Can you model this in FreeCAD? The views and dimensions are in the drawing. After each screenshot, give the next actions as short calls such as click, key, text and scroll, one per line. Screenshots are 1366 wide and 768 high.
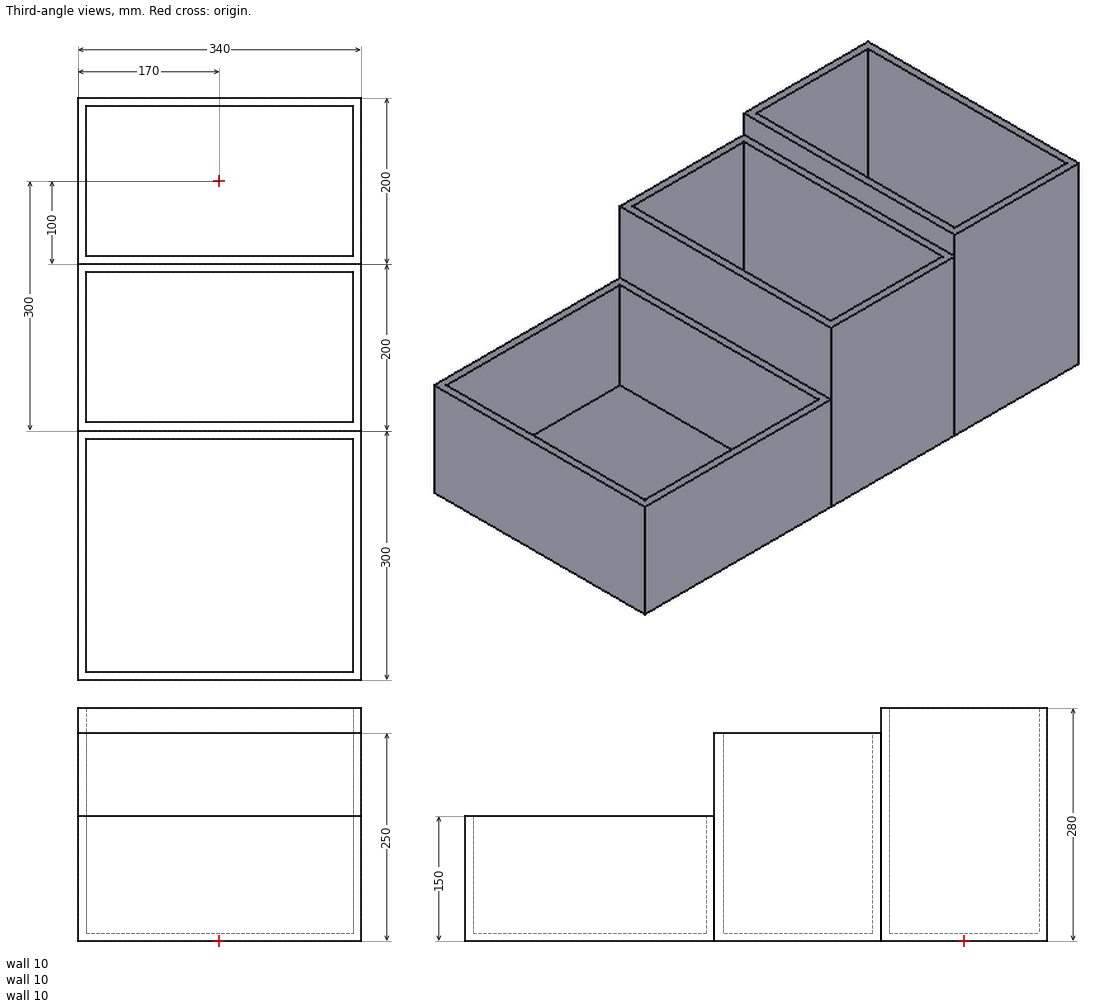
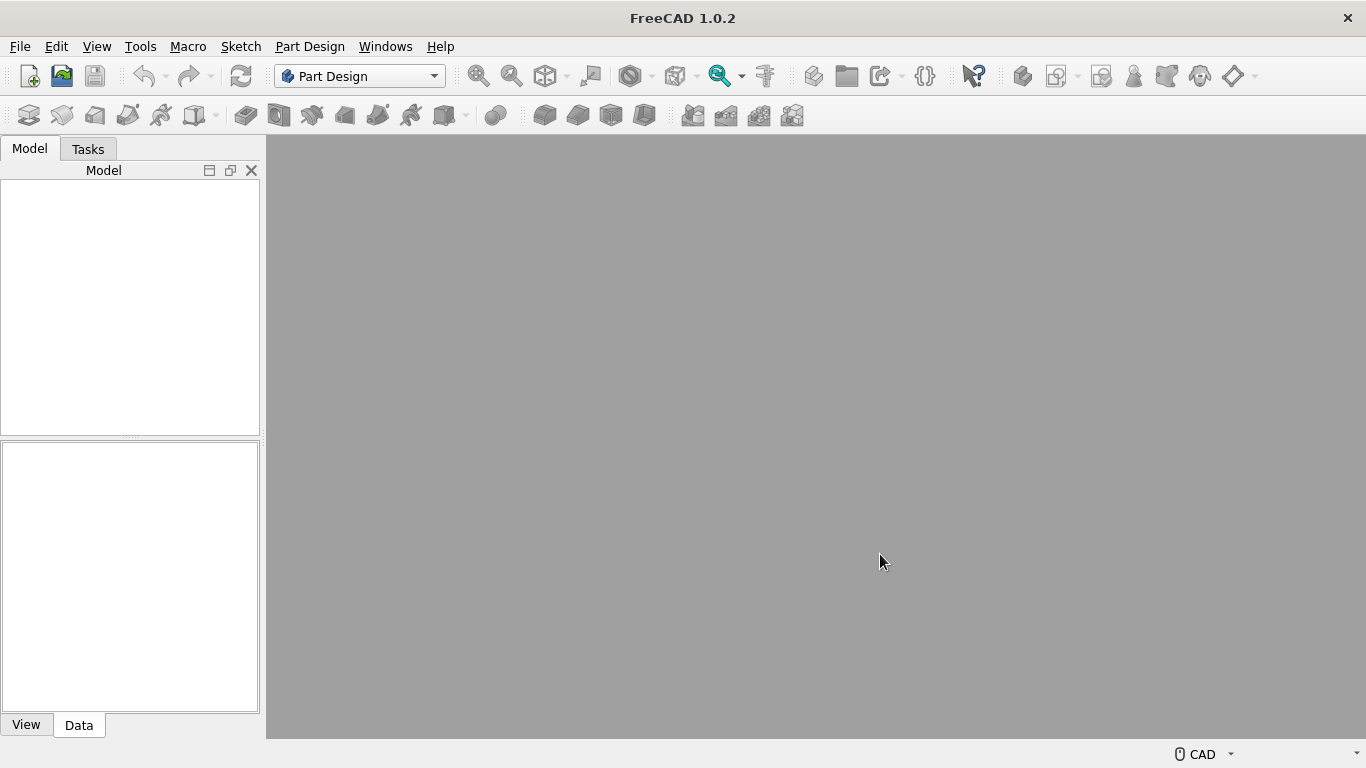
key(ctrl+n)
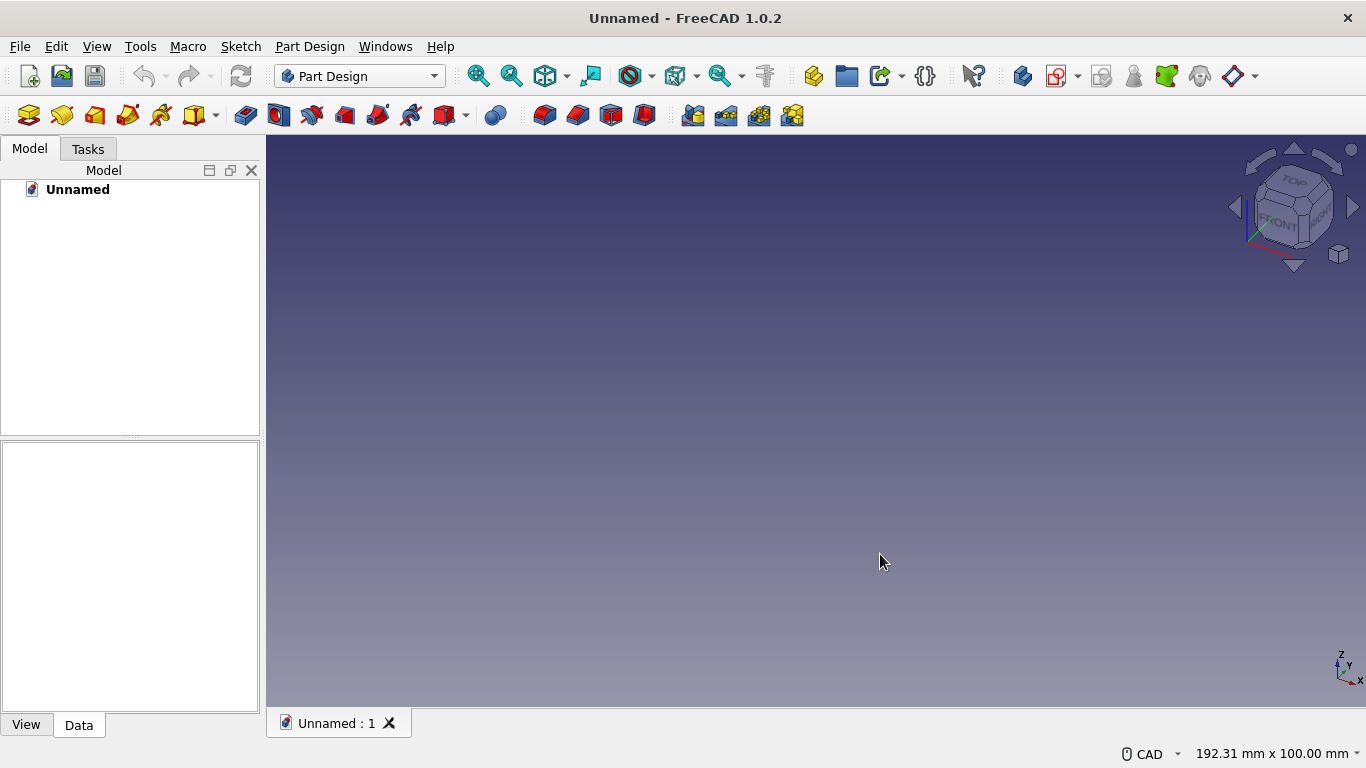
click(1056, 76)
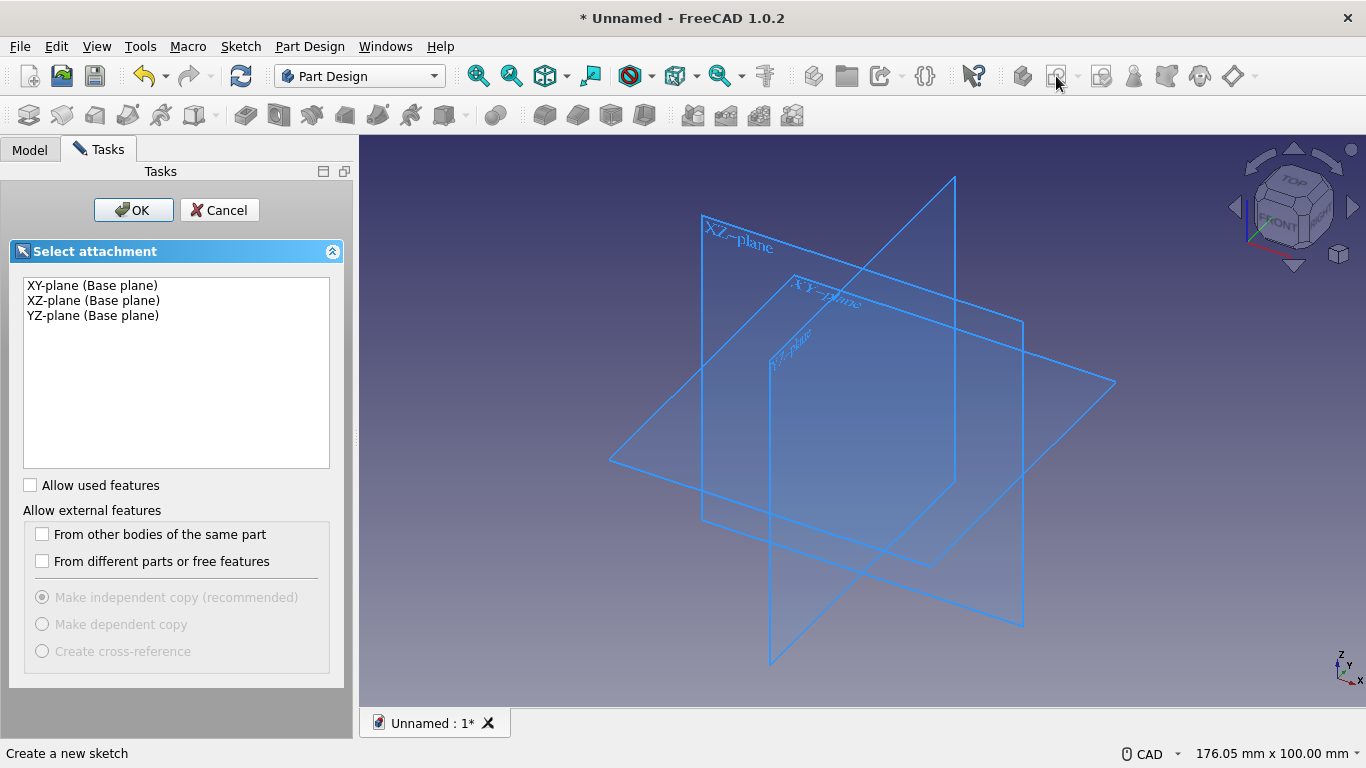
click(84, 286)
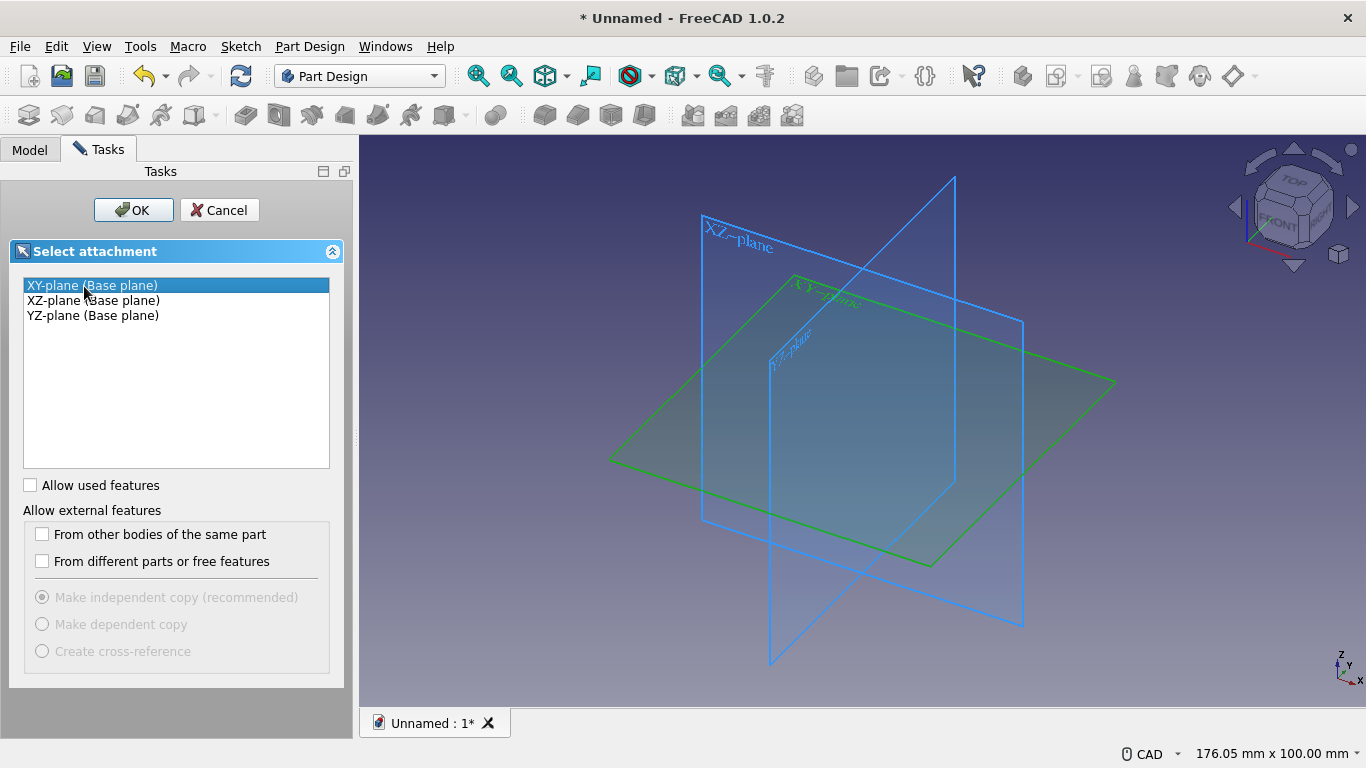
click(134, 210)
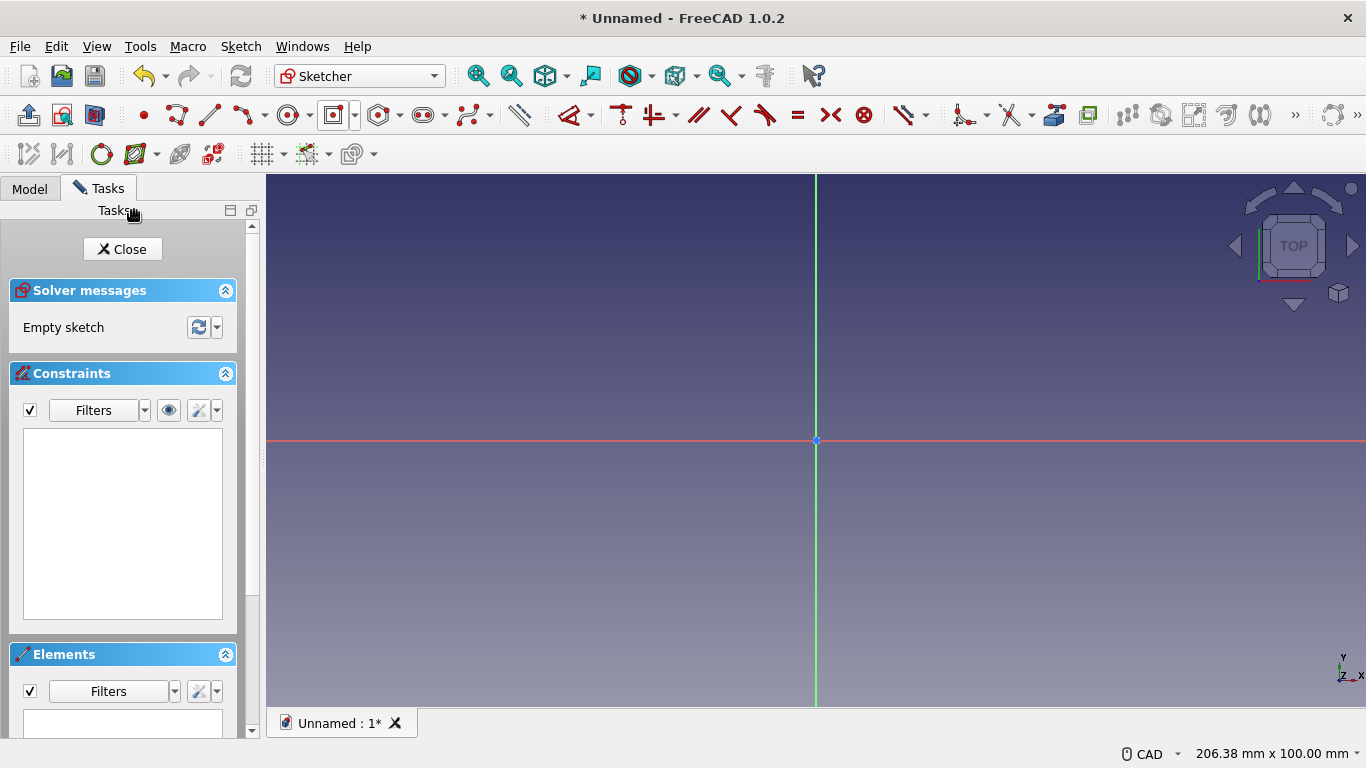
scroll(718, 440, down, 6)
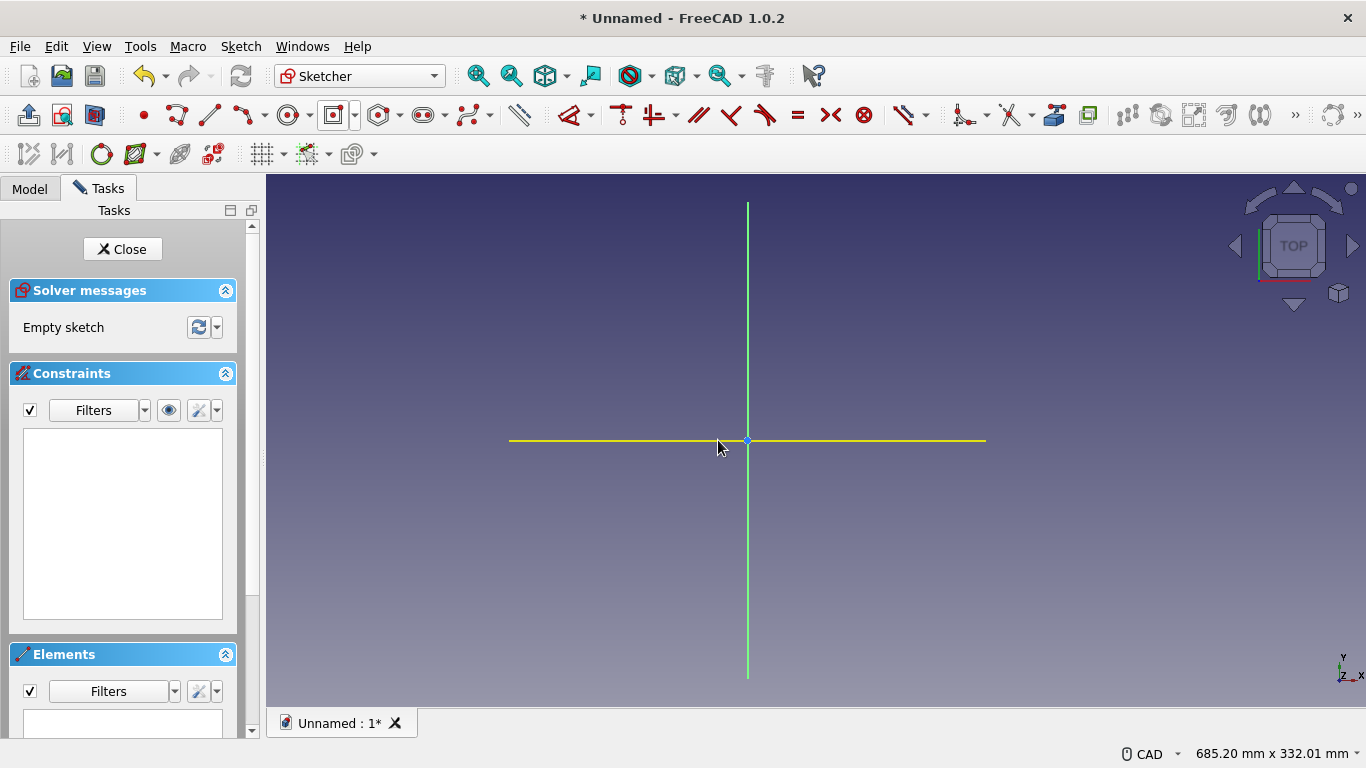
click(332, 116)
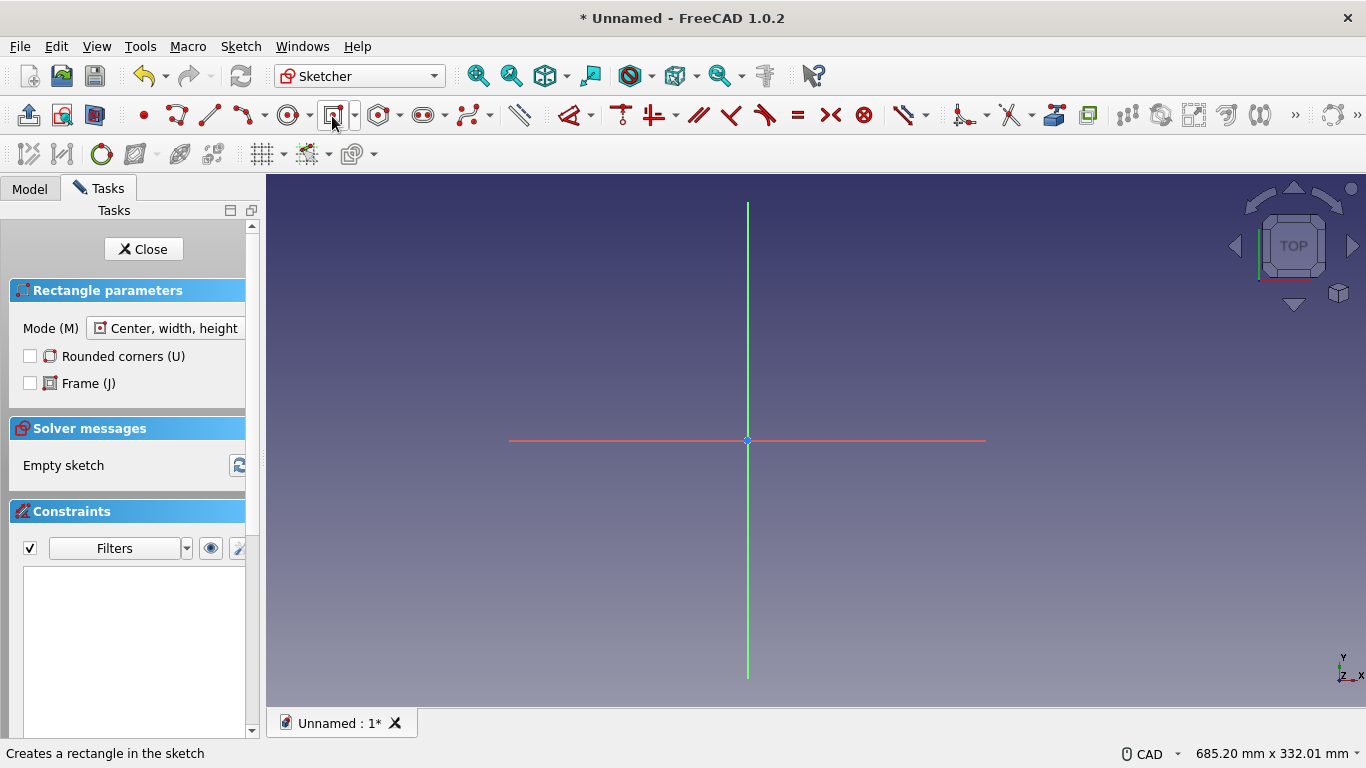
click(748, 440)
move(1021, 280)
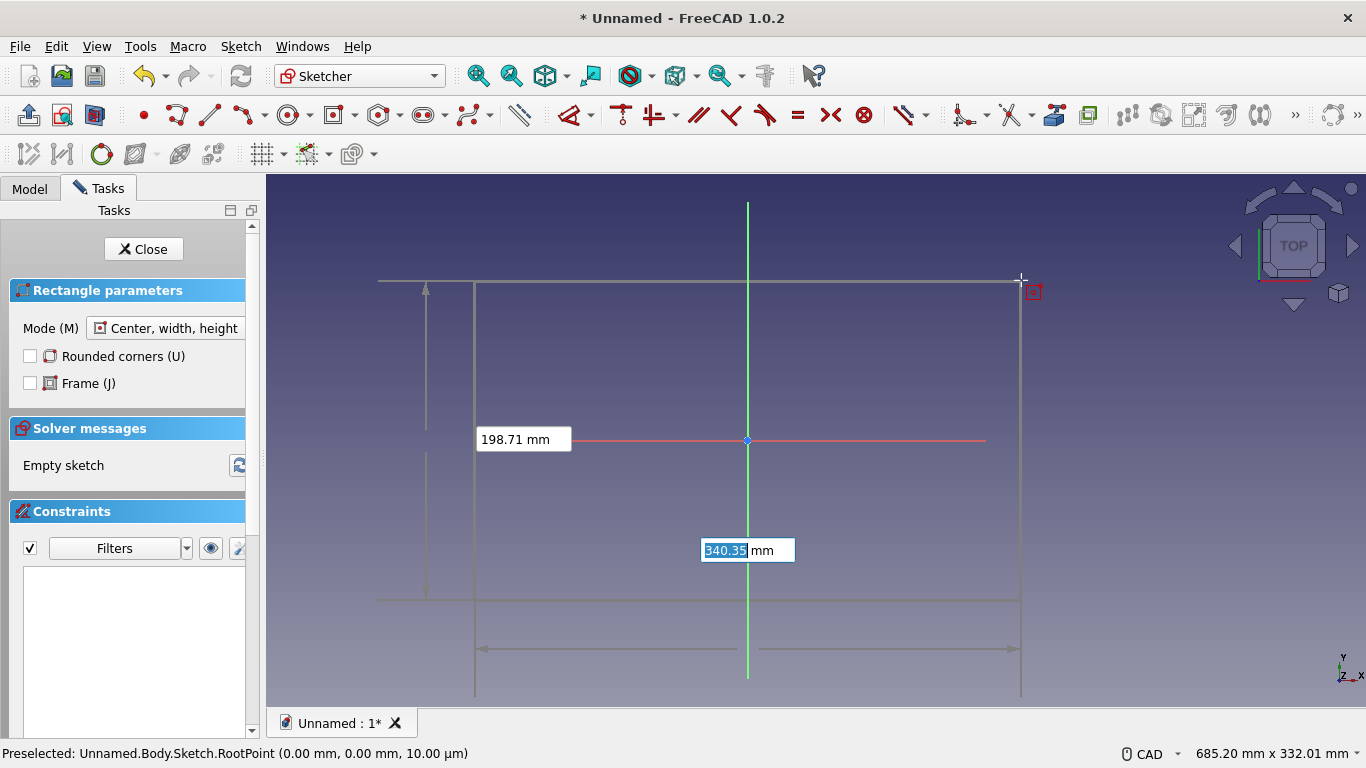
text(340)
key(Tab)
text(200)
key(Return)
key(Escape)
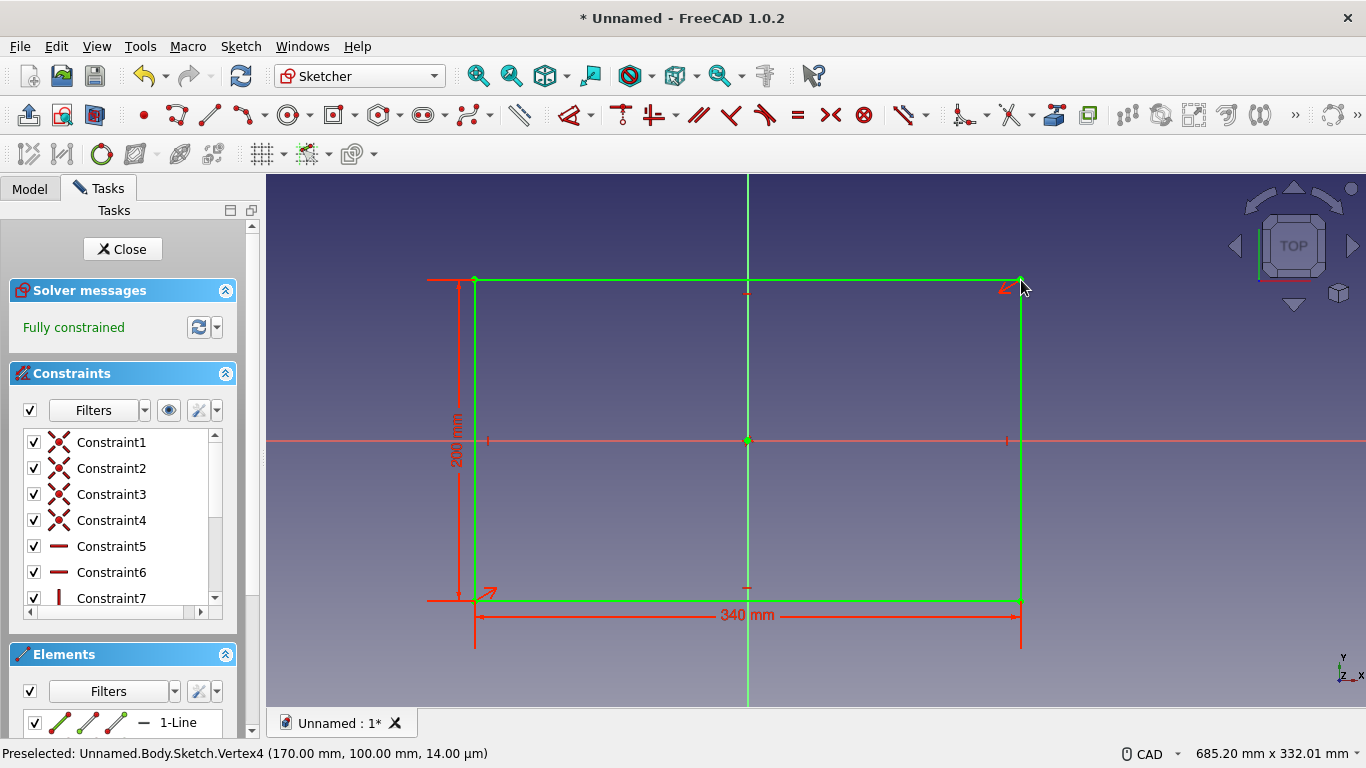
click(123, 249)